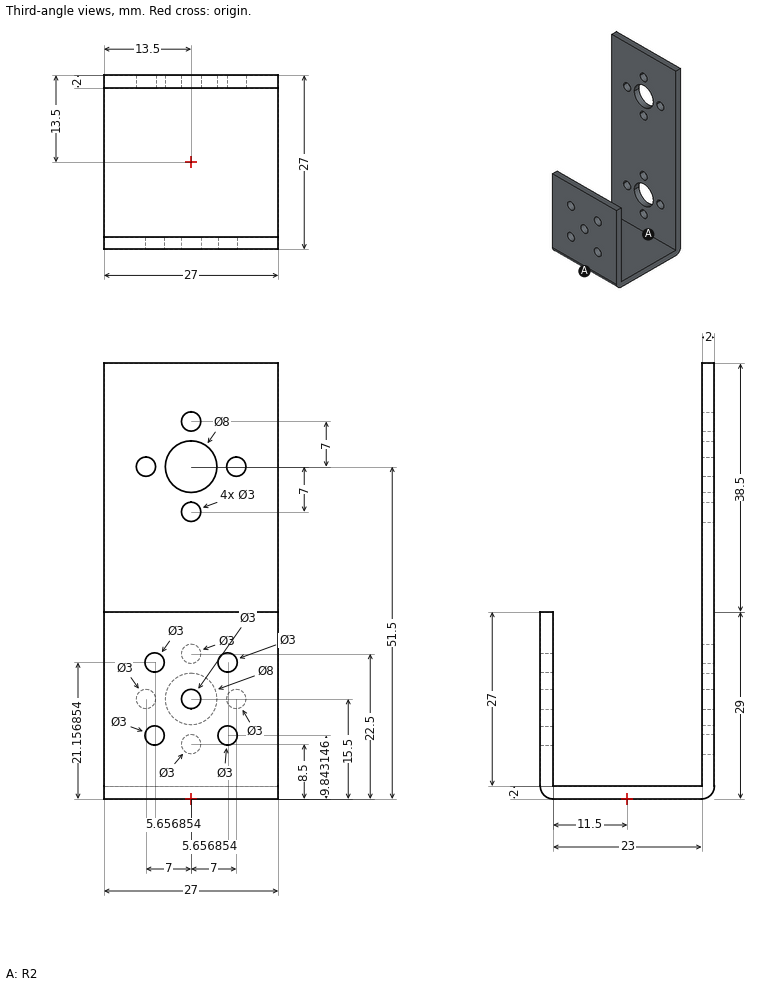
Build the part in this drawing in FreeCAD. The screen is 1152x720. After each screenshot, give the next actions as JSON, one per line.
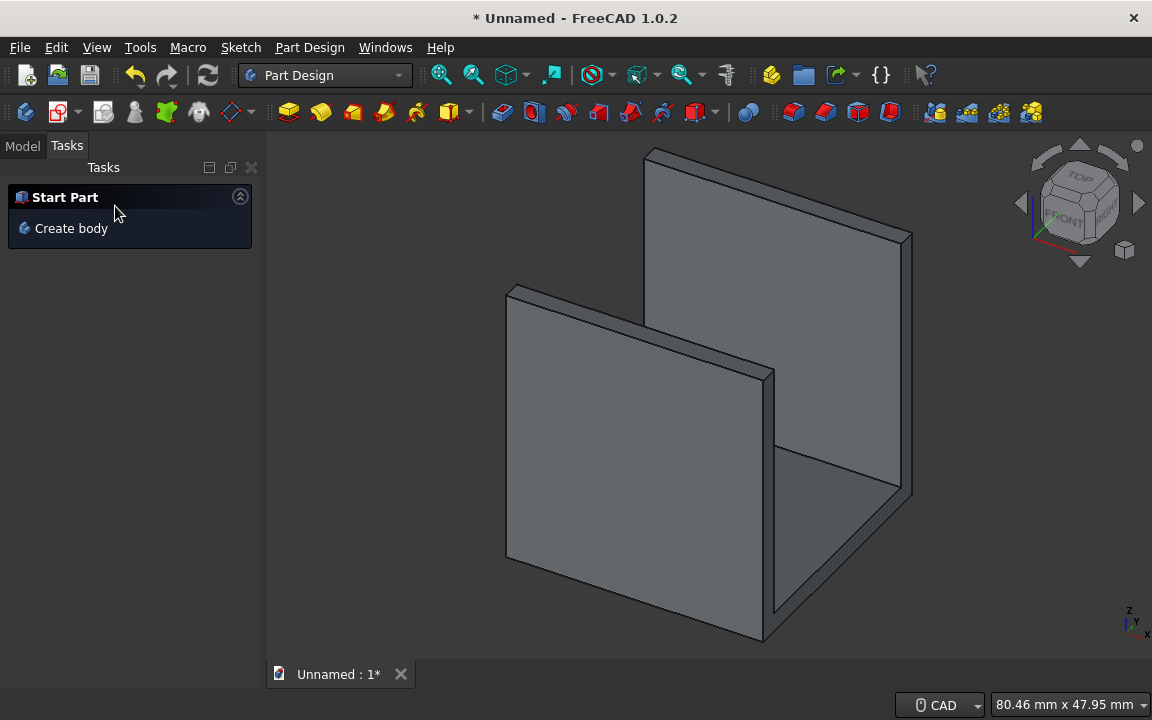
{"action": "key", "text": "4"}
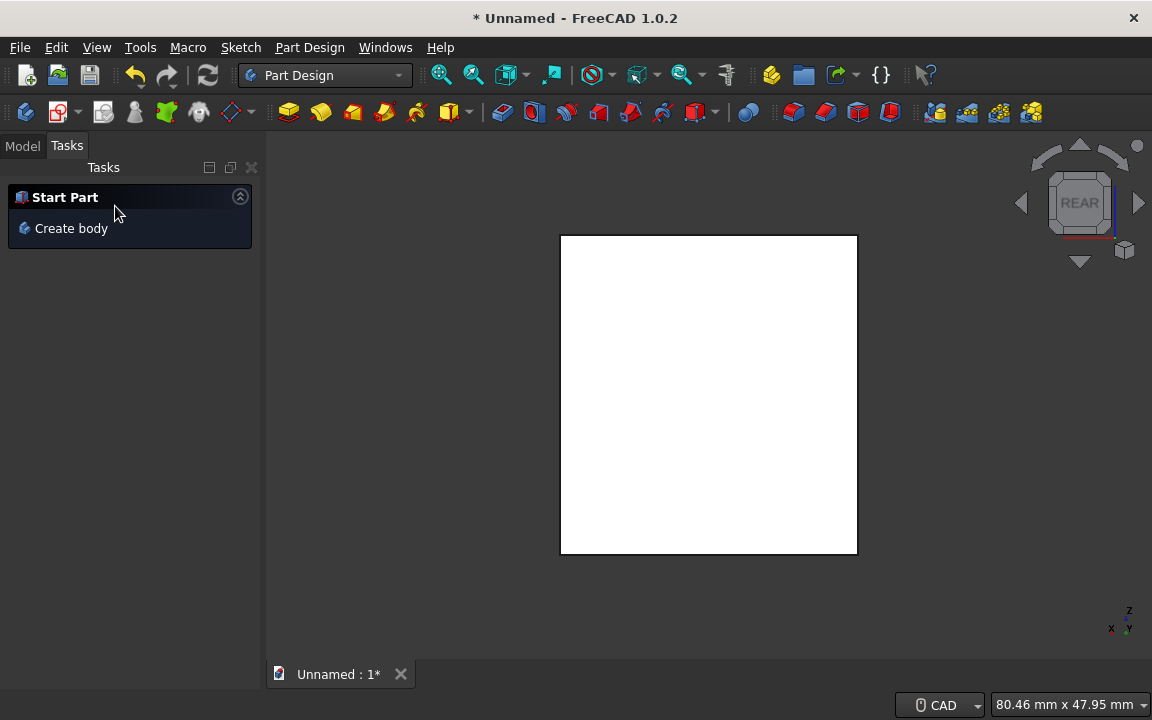
{"action": "left_click", "coordinate": [709, 394]}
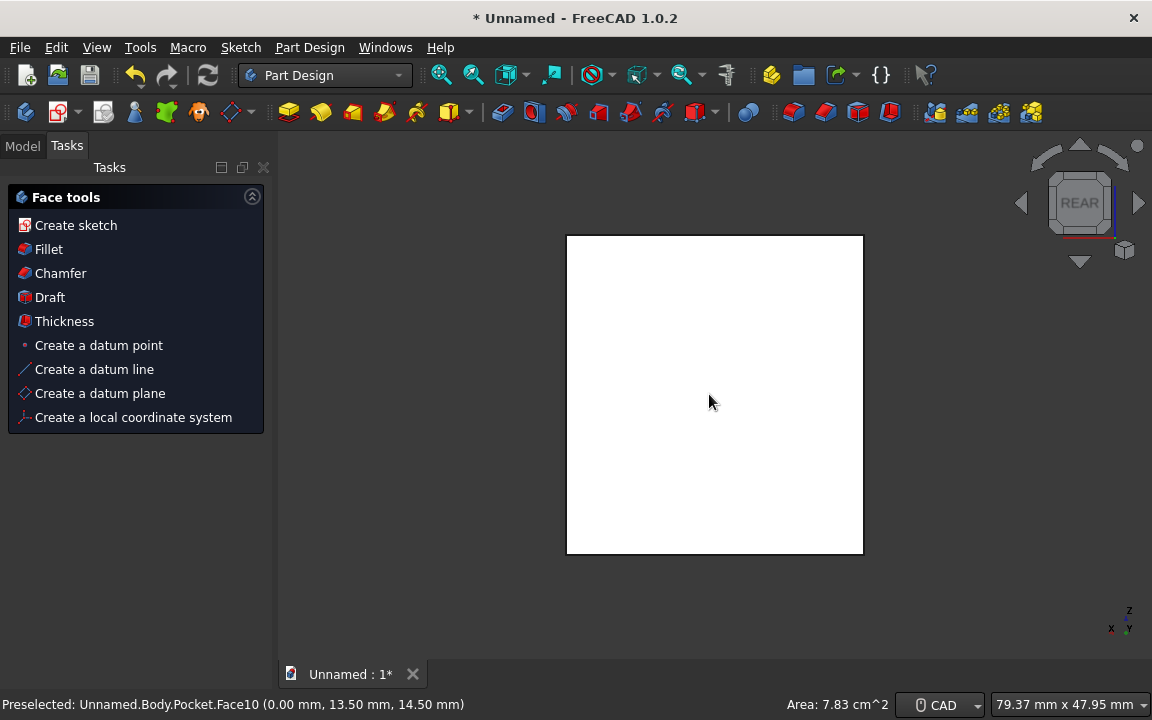
{"action": "left_click", "coordinate": [58, 112]}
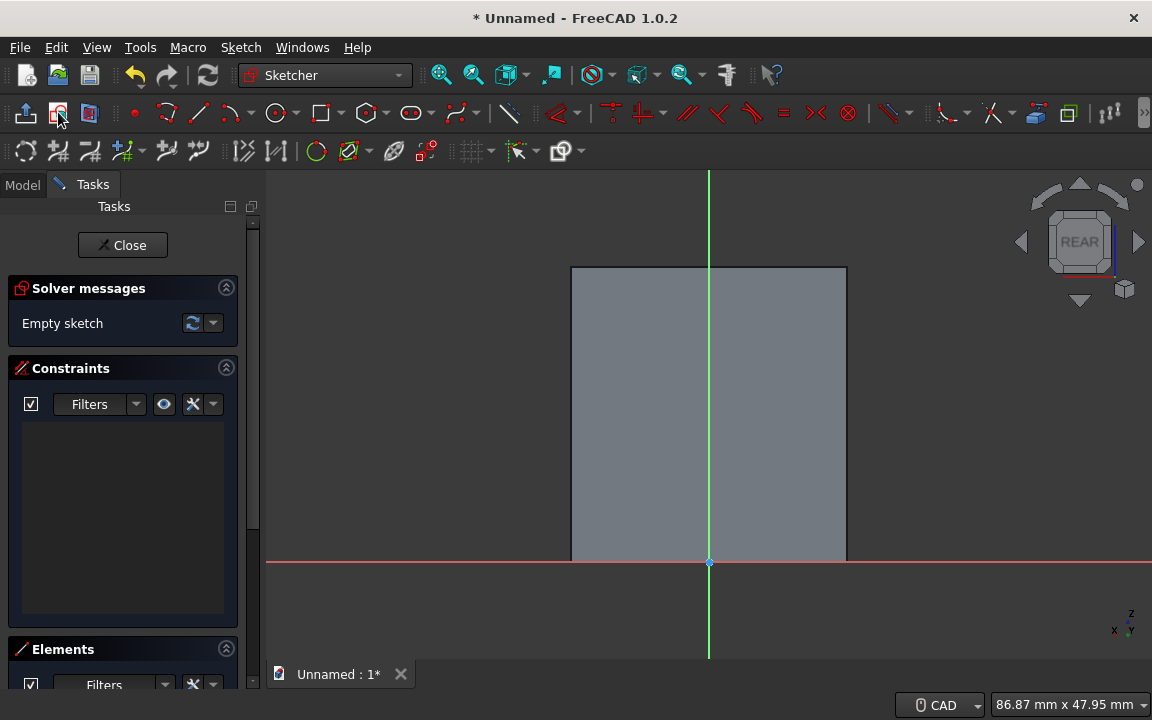
{"action": "scroll", "coordinate": [848, 561], "scroll_direction": "up", "scroll_amount": 2}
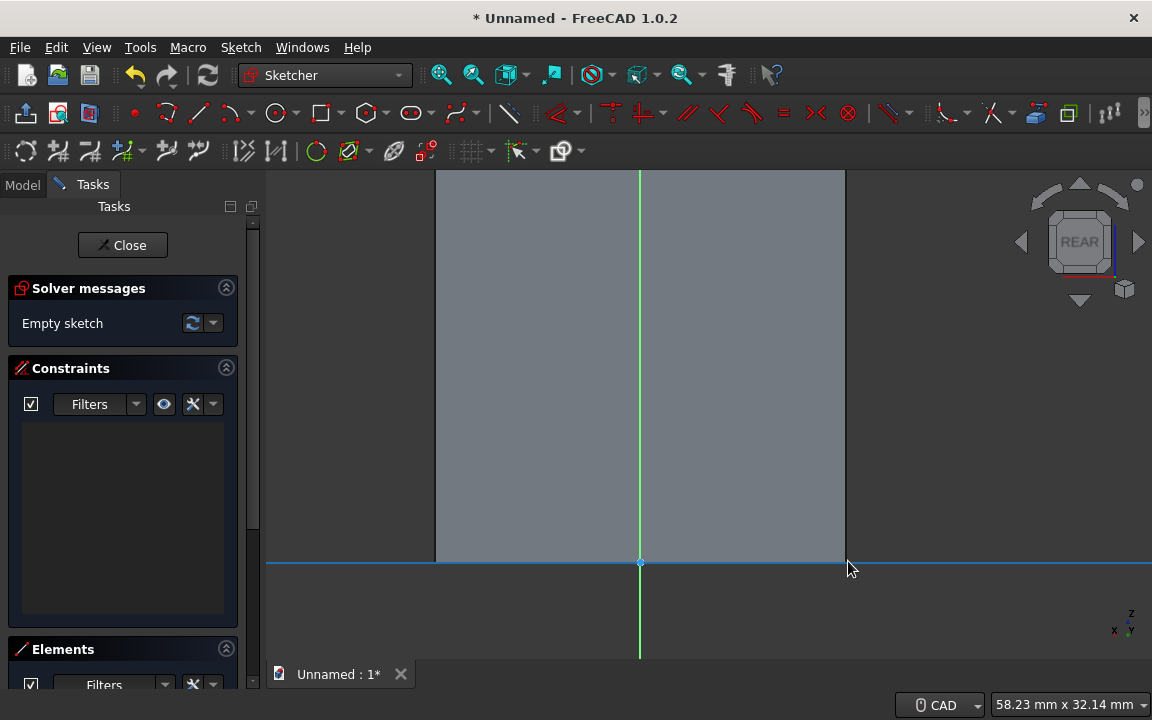
{"action": "left_click", "coordinate": [276, 114]}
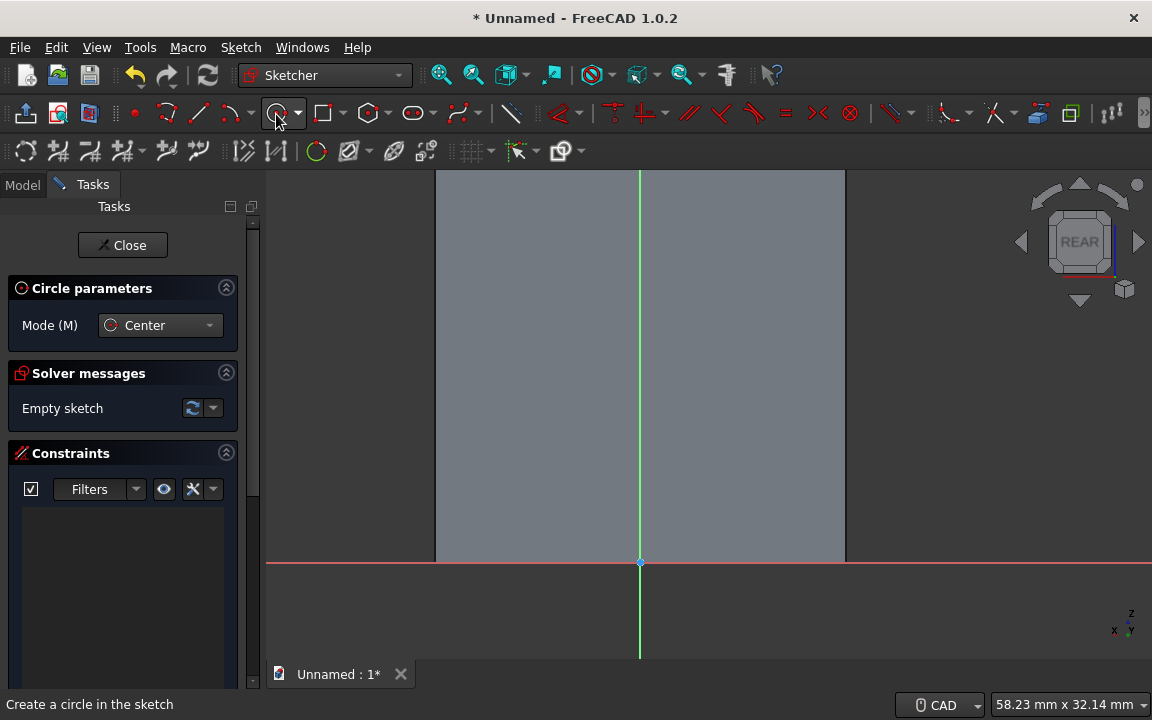
{"action": "left_click", "coordinate": [640, 327]}
{"action": "left_click", "coordinate": [683, 284]}
{"action": "key", "text": "Escape"}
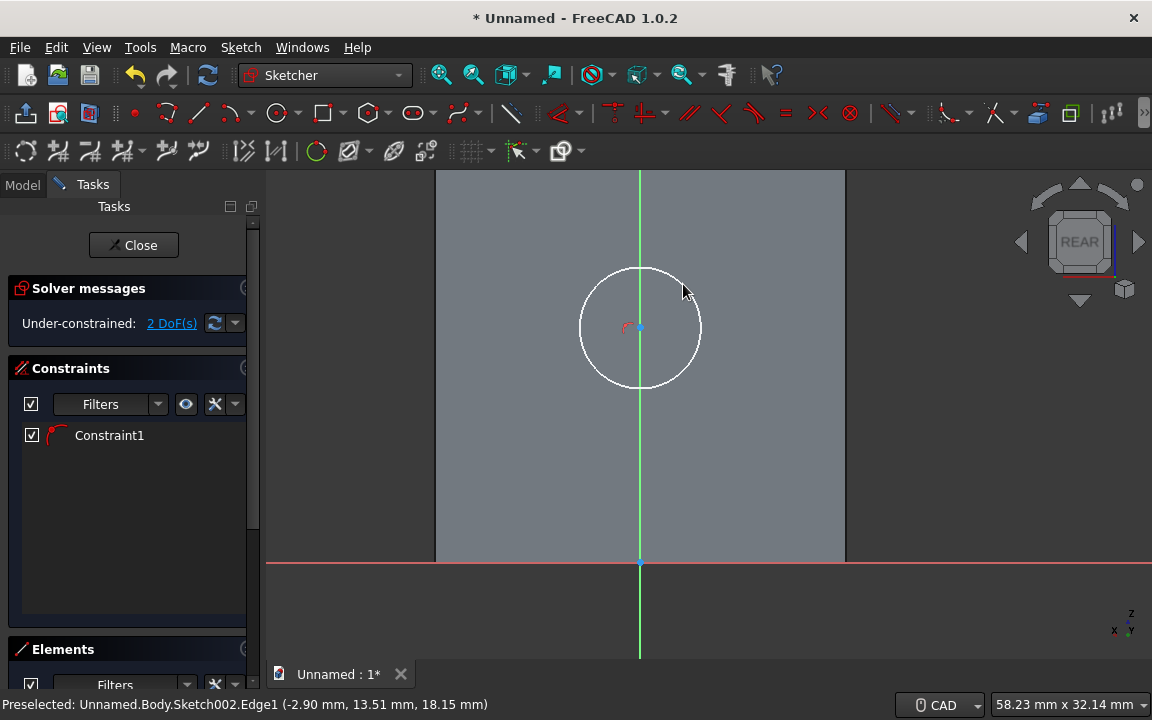
{"action": "key", "text": "d"}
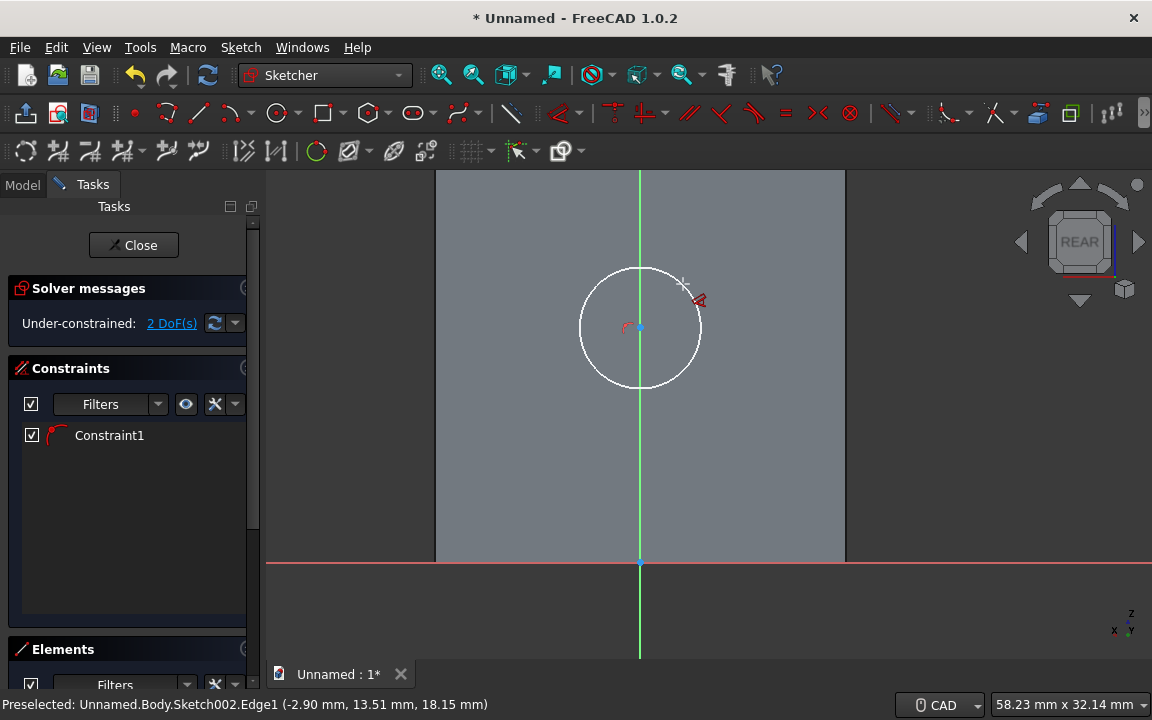
{"action": "left_click", "coordinate": [683, 285]}
{"action": "left_click", "coordinate": [706, 262]}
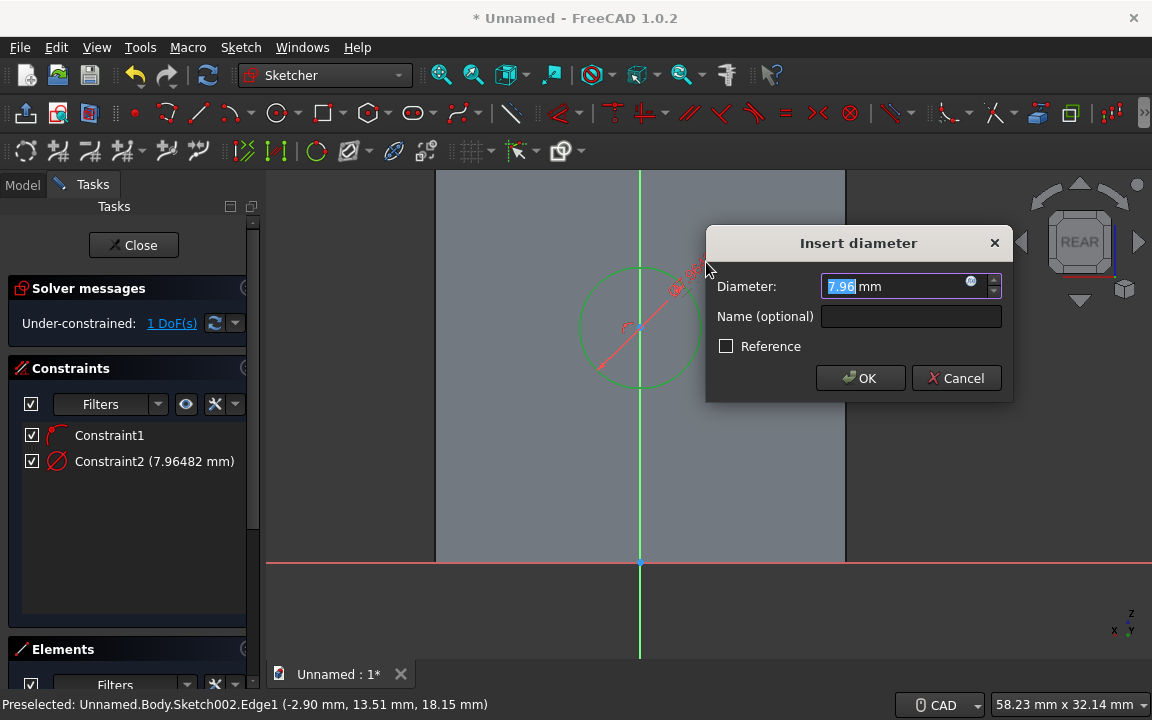
{"action": "type", "text": "8"}
{"action": "key", "text": "Return"}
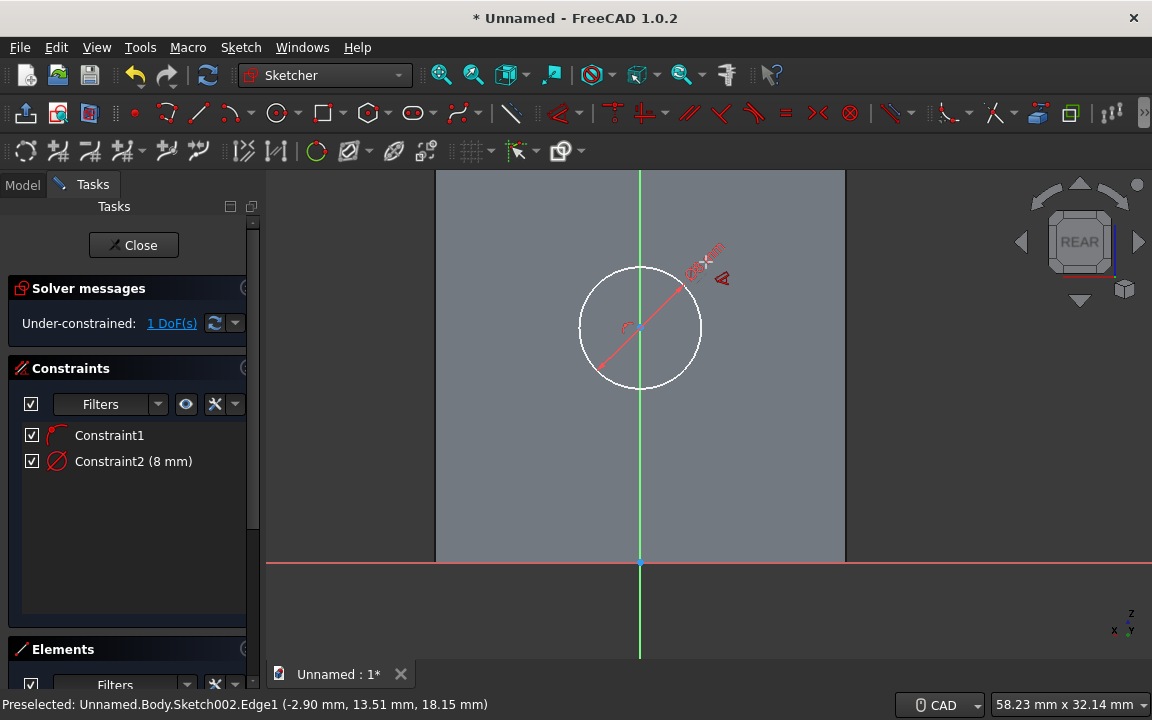
{"action": "left_click", "coordinate": [640, 328]}
{"action": "left_click", "coordinate": [674, 445]}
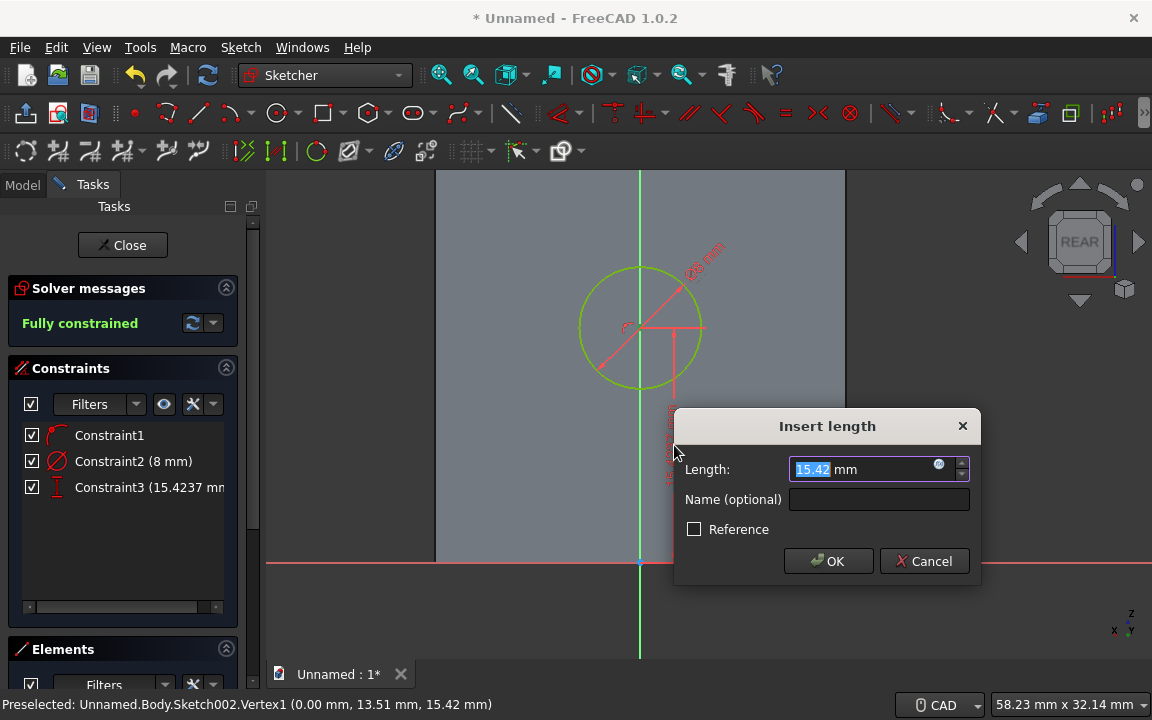
{"action": "type", "text": "15.5"}
{"action": "key", "text": "Return"}
{"action": "key", "text": "Escape"}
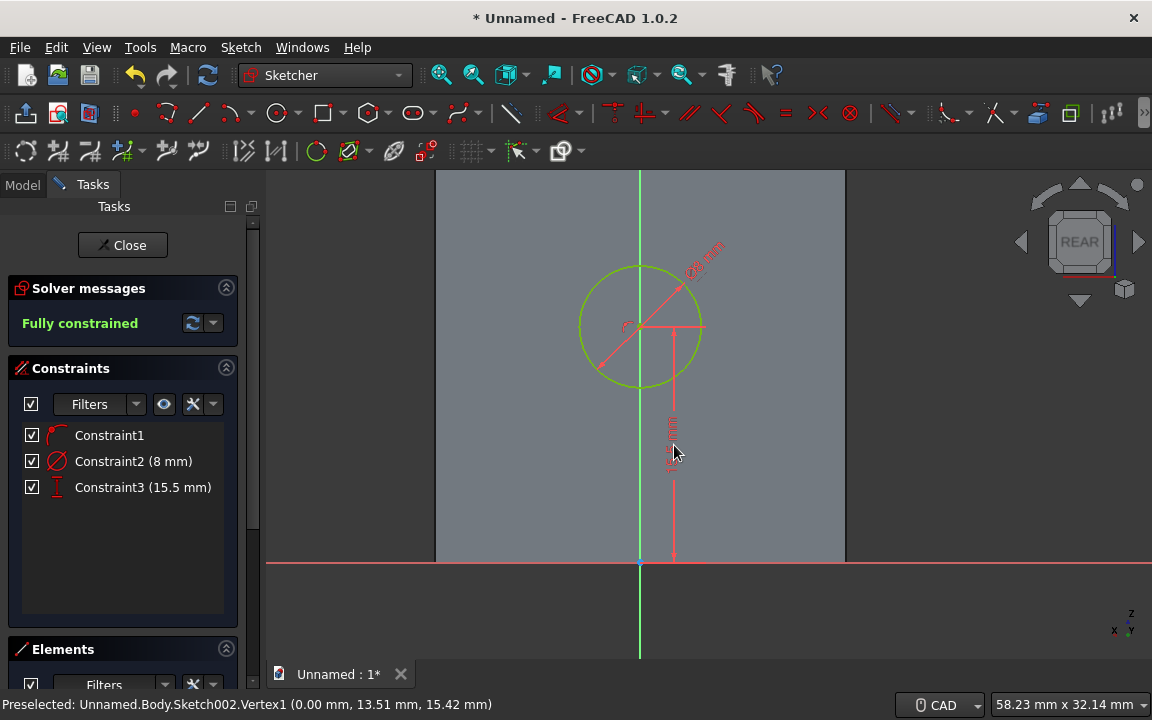
{"action": "left_click", "coordinate": [123, 245]}